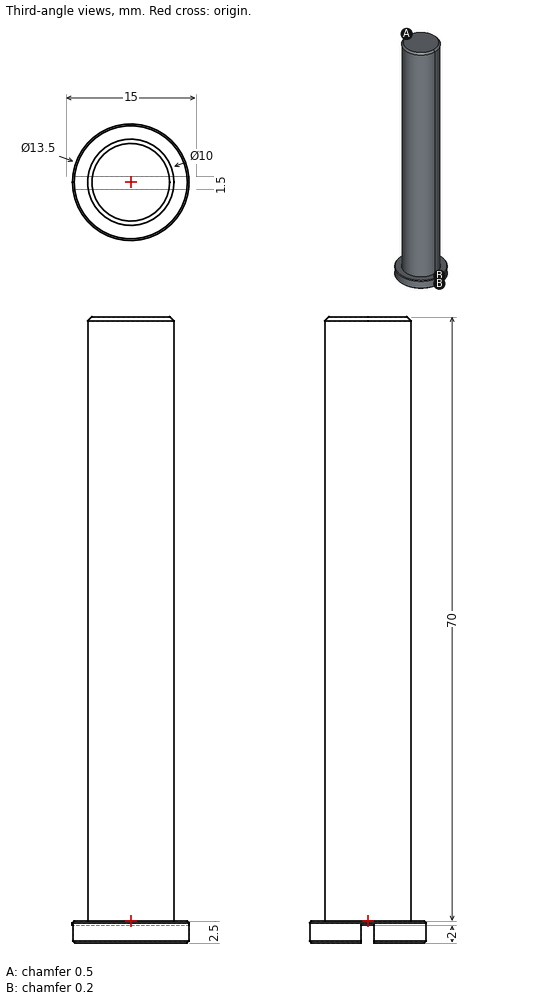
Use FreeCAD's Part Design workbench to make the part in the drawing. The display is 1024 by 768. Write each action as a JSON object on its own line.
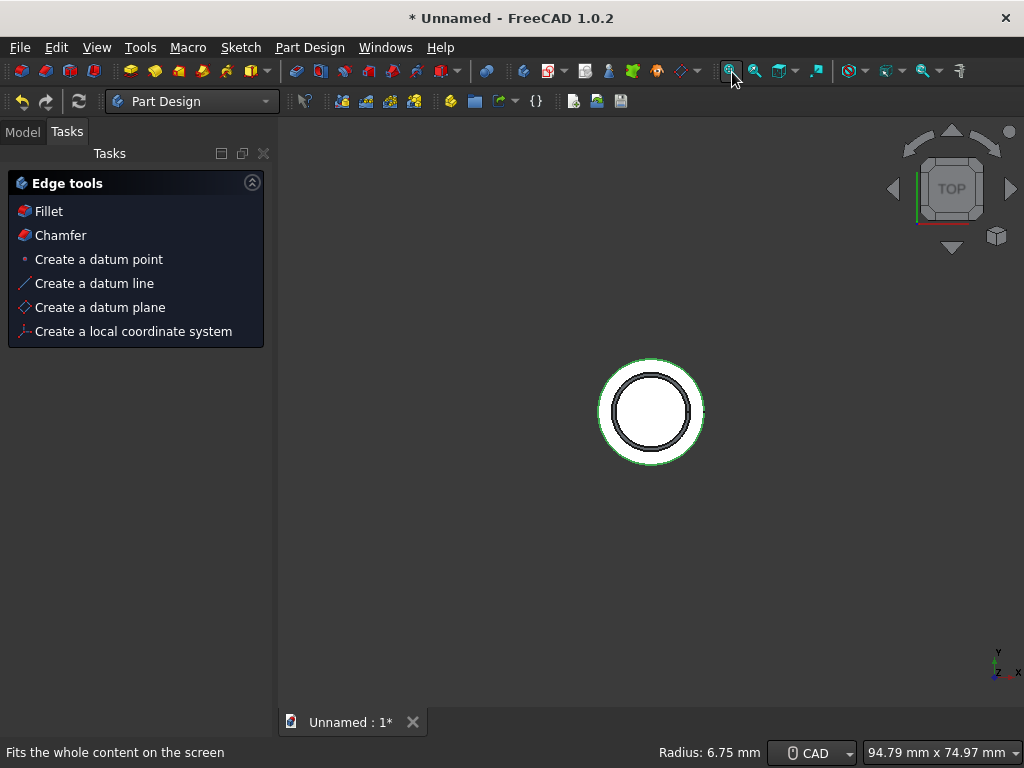
{"action": "key", "text": "1"}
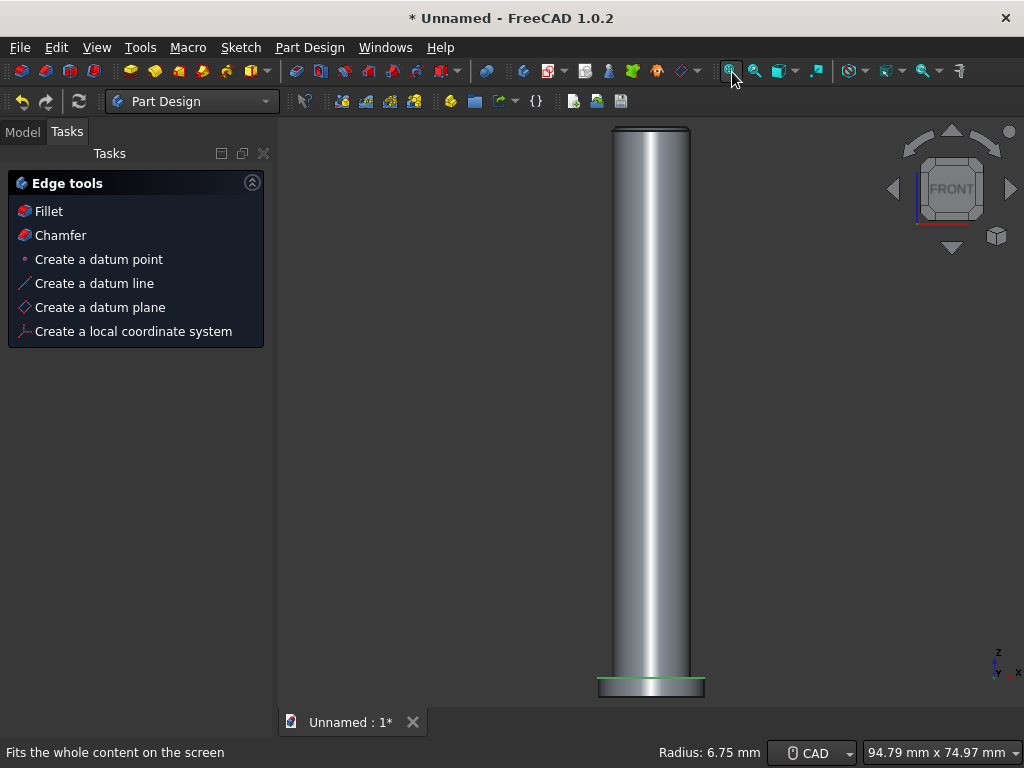
{"action": "key", "text": "3"}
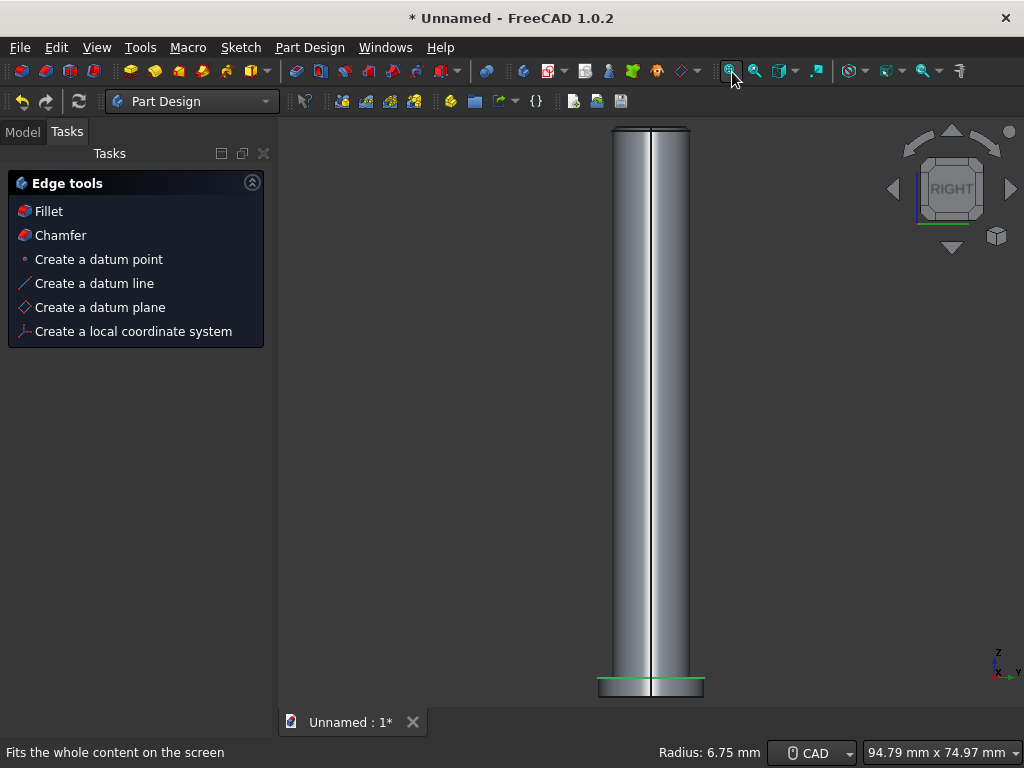
{"action": "key", "text": "5"}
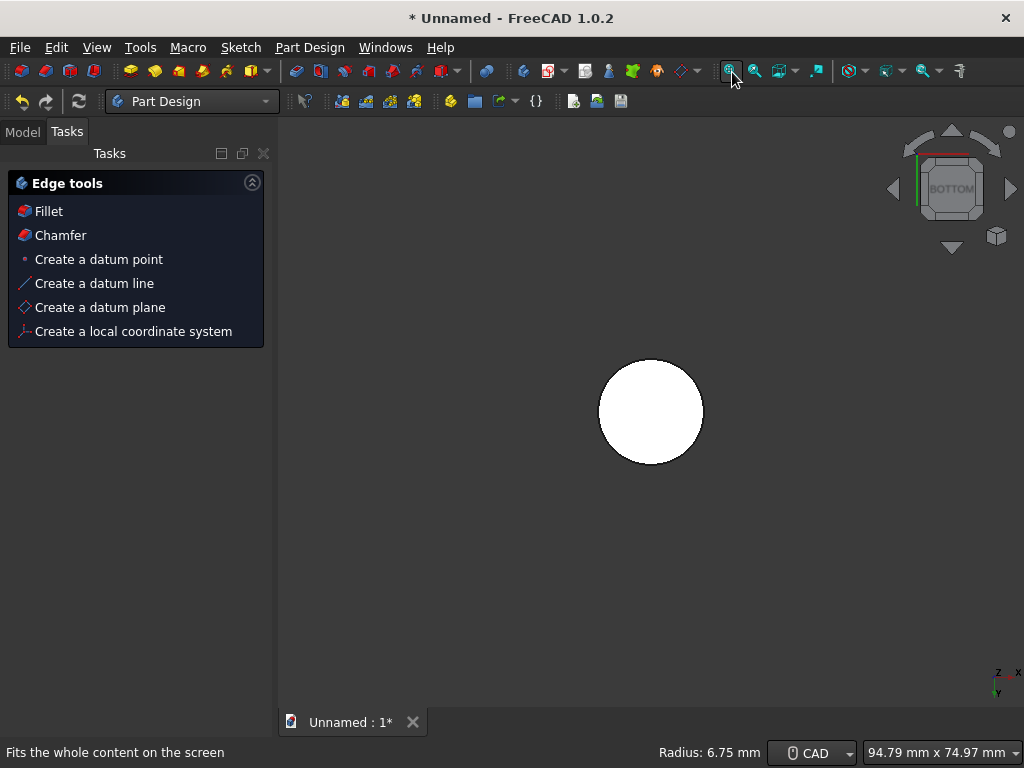
{"action": "left_click", "coordinate": [732, 72]}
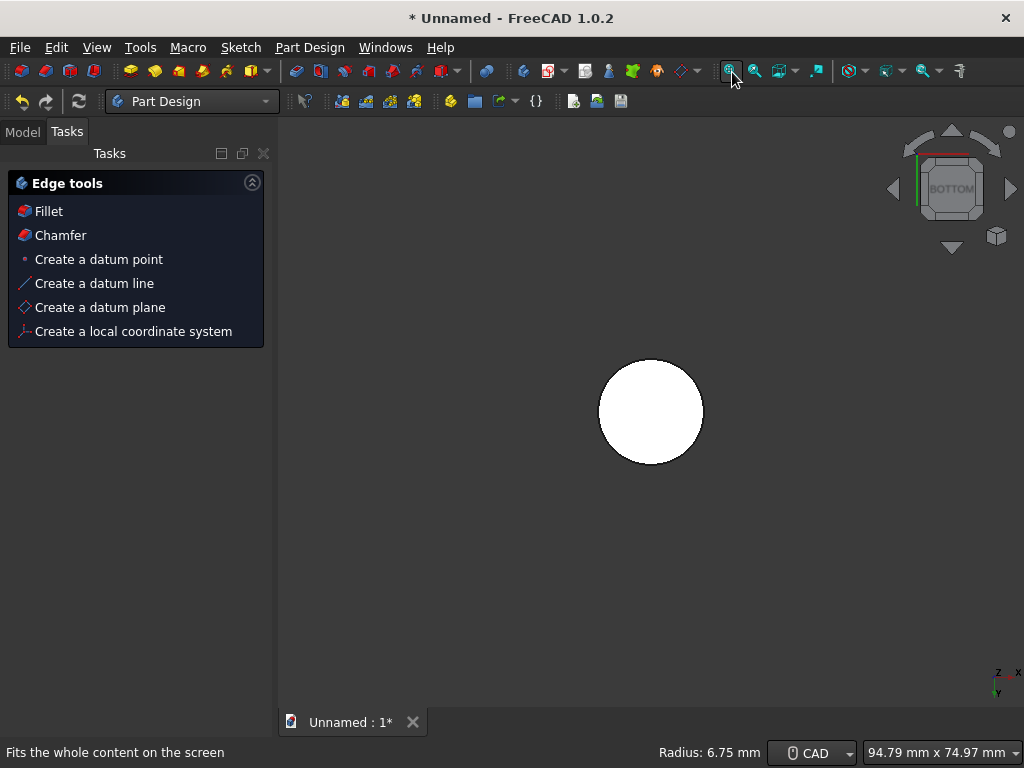
{"action": "left_click", "coordinate": [598, 411], "text": "ctrl"}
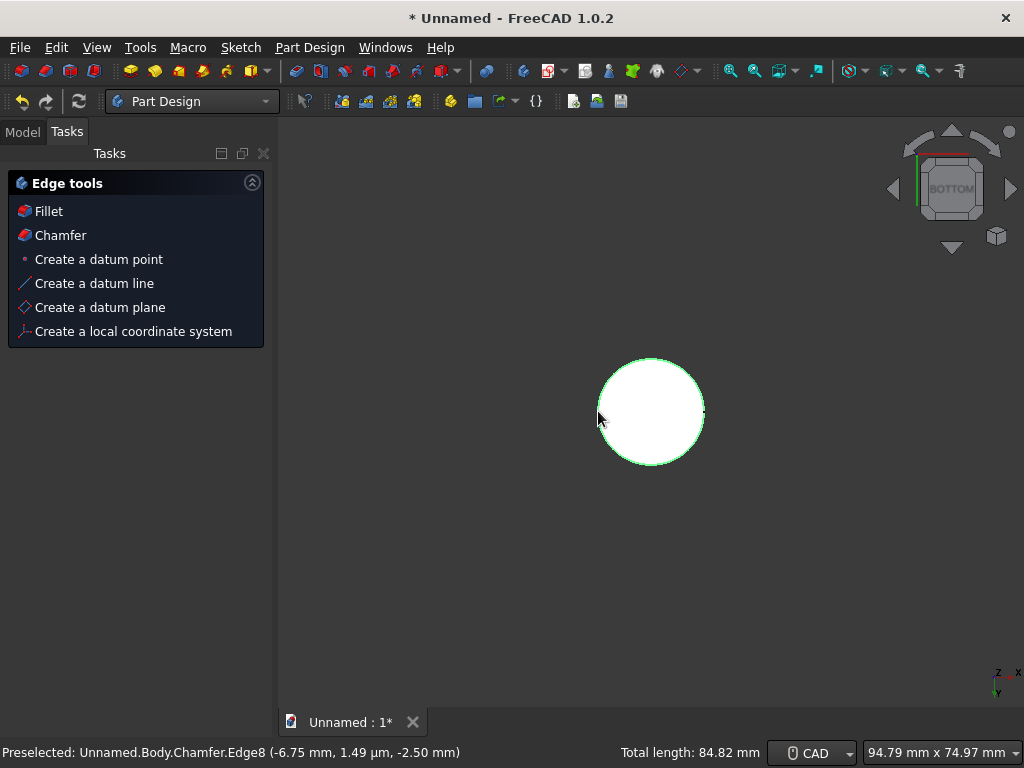
{"action": "left_click", "coordinate": [46, 72]}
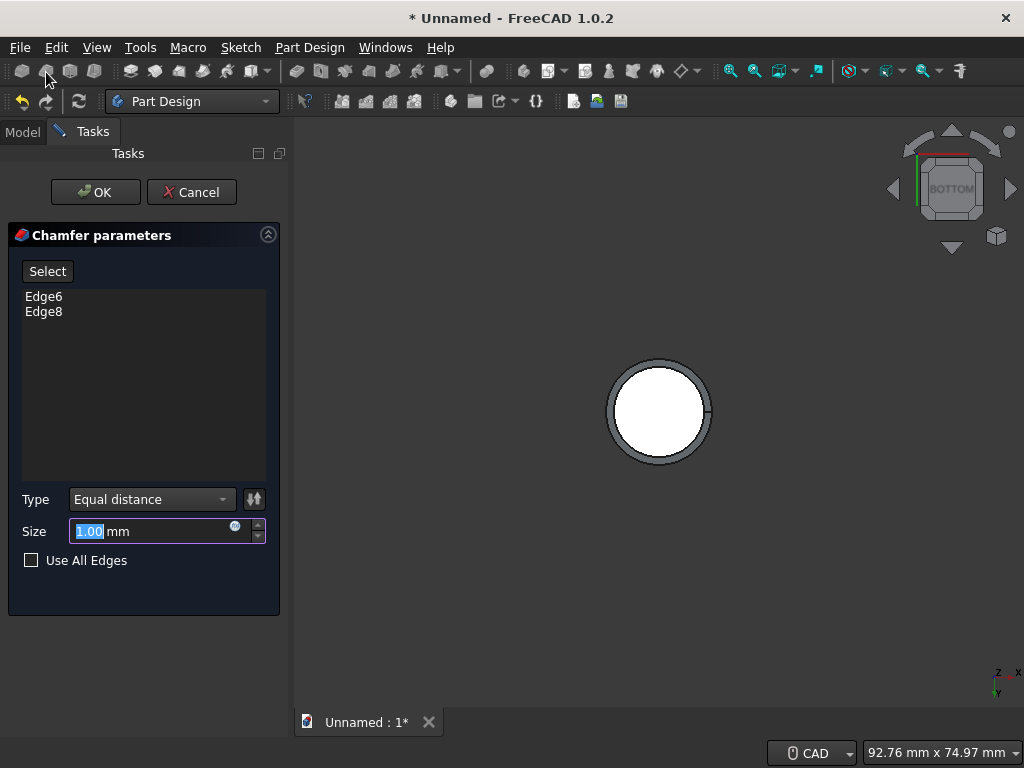
{"action": "type", "text": "0.2"}
{"action": "key", "text": "Tab"}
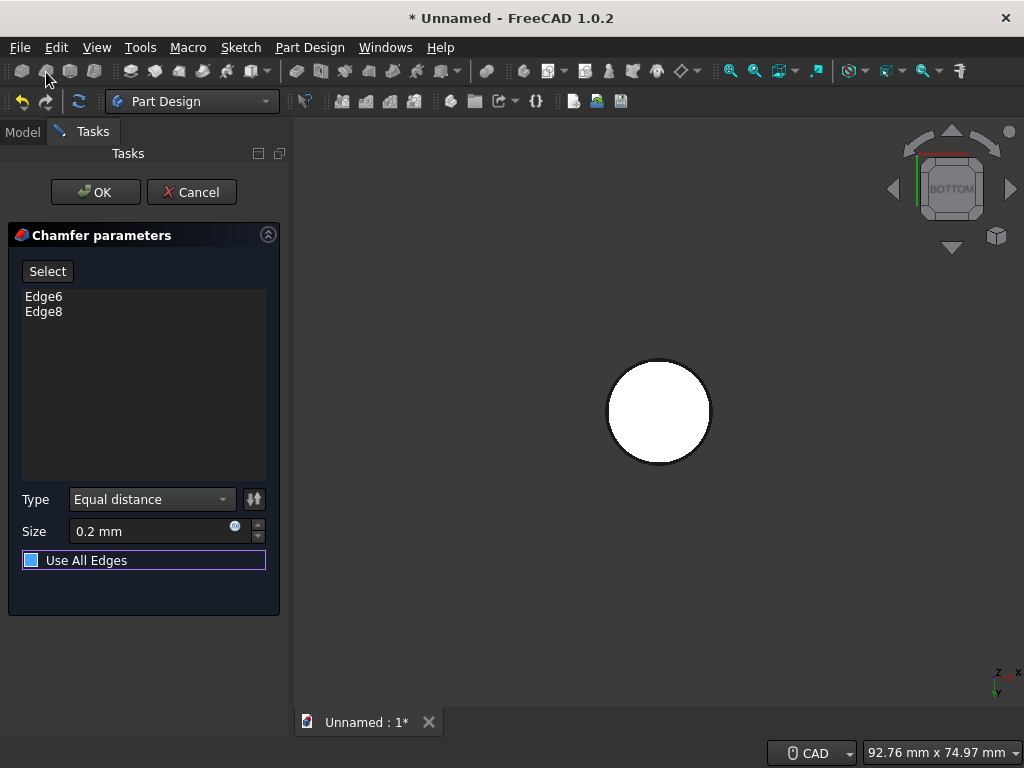
{"action": "left_click", "coordinate": [96, 192]}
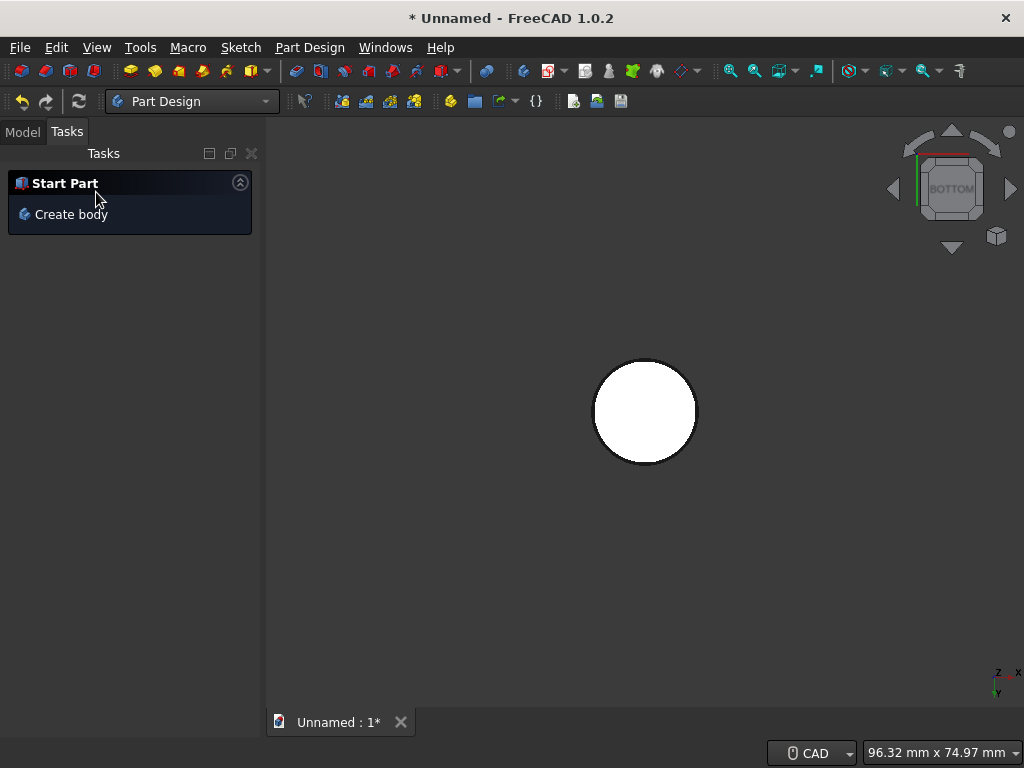
{"action": "left_click", "coordinate": [732, 72]}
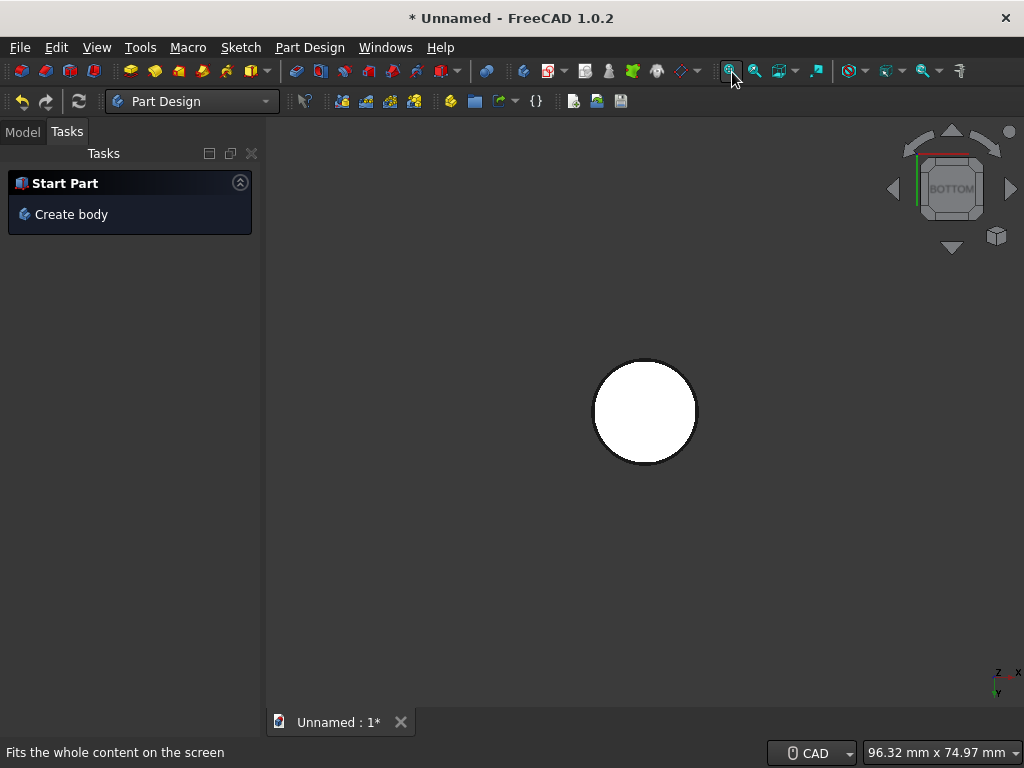
{"action": "left_click", "coordinate": [645, 411]}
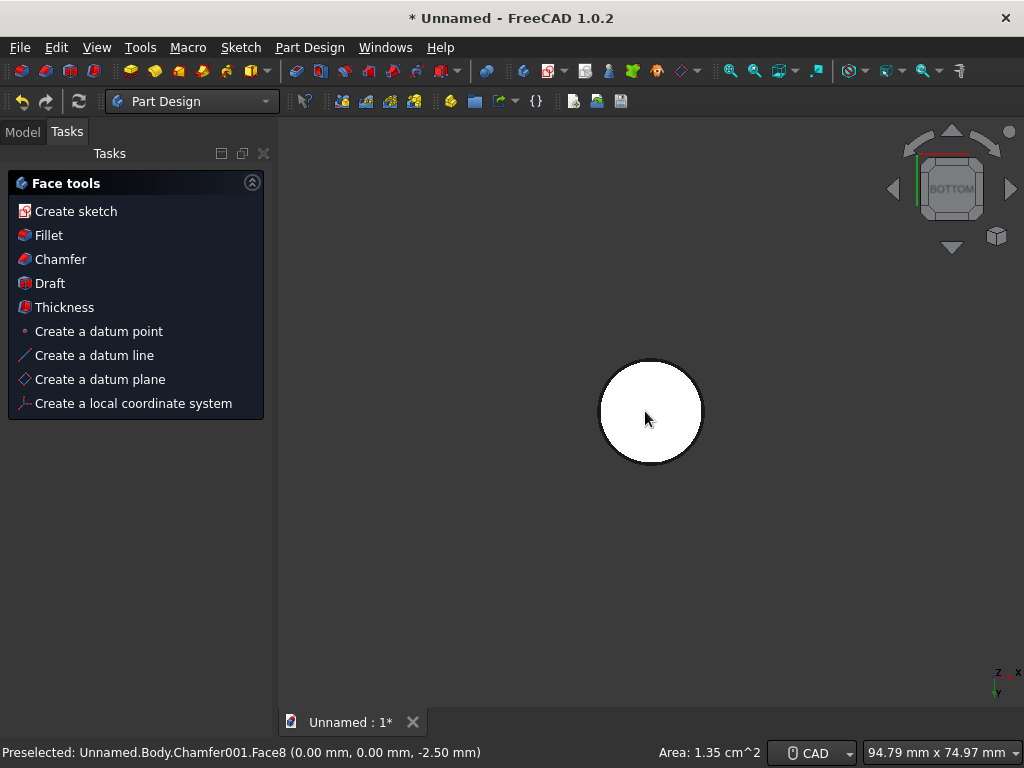
{"action": "left_click", "coordinate": [548, 72]}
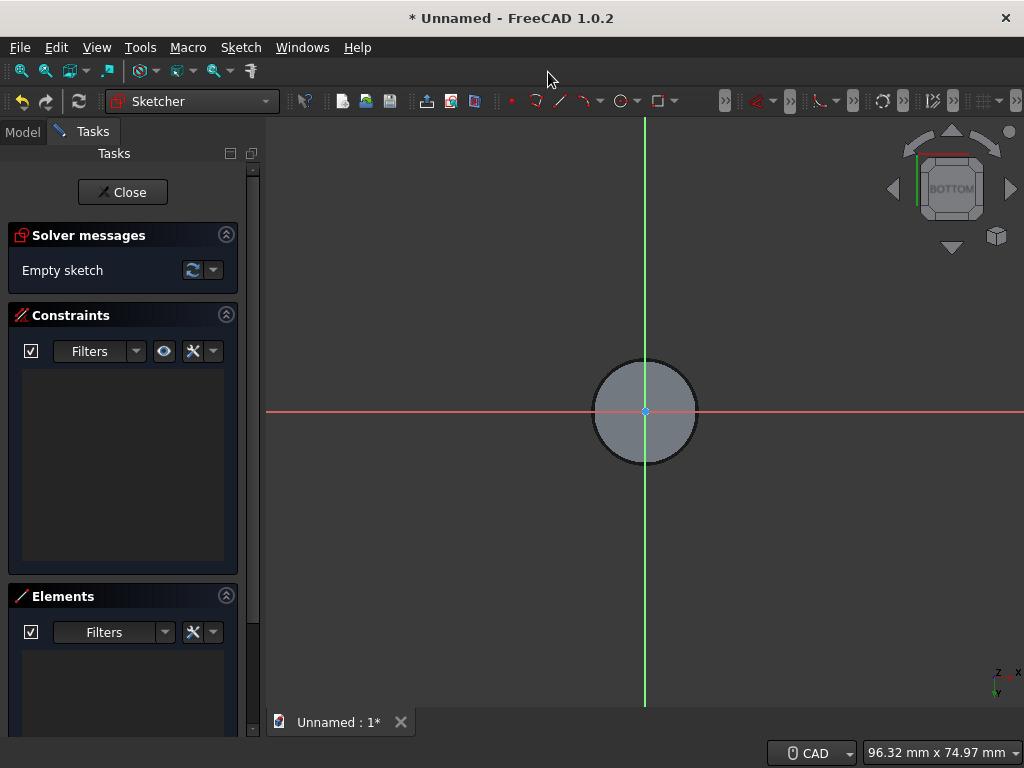
{"action": "scroll", "coordinate": [675, 412], "scroll_direction": "up", "scroll_amount": 6}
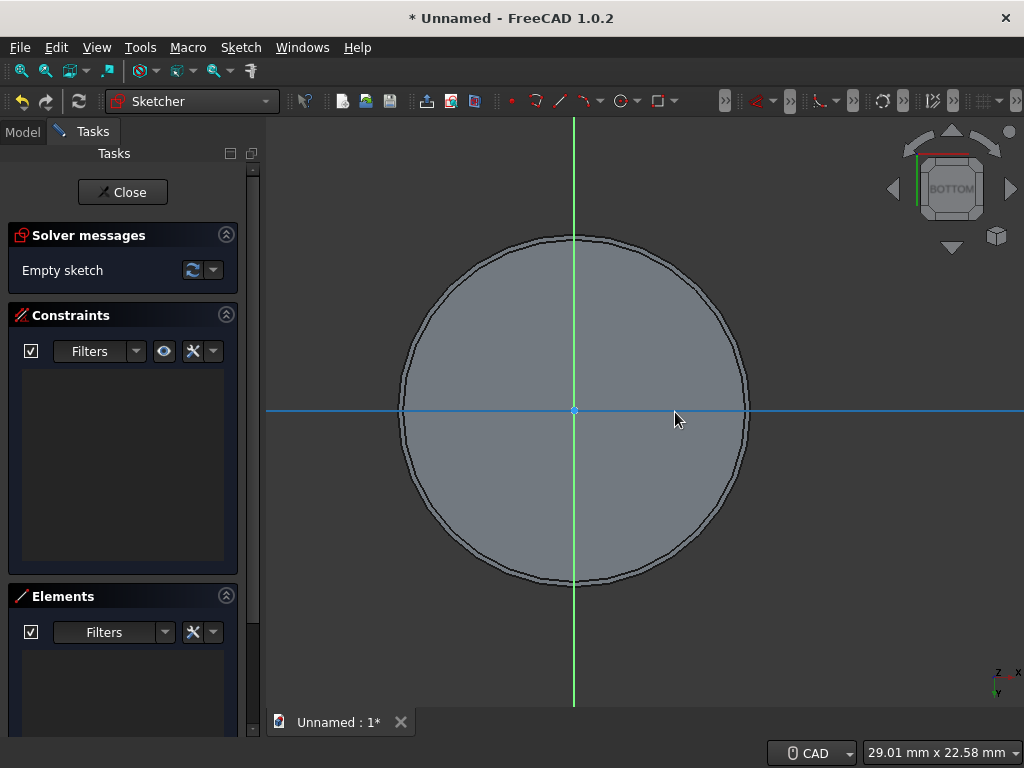
{"action": "left_click", "coordinate": [676, 102]}